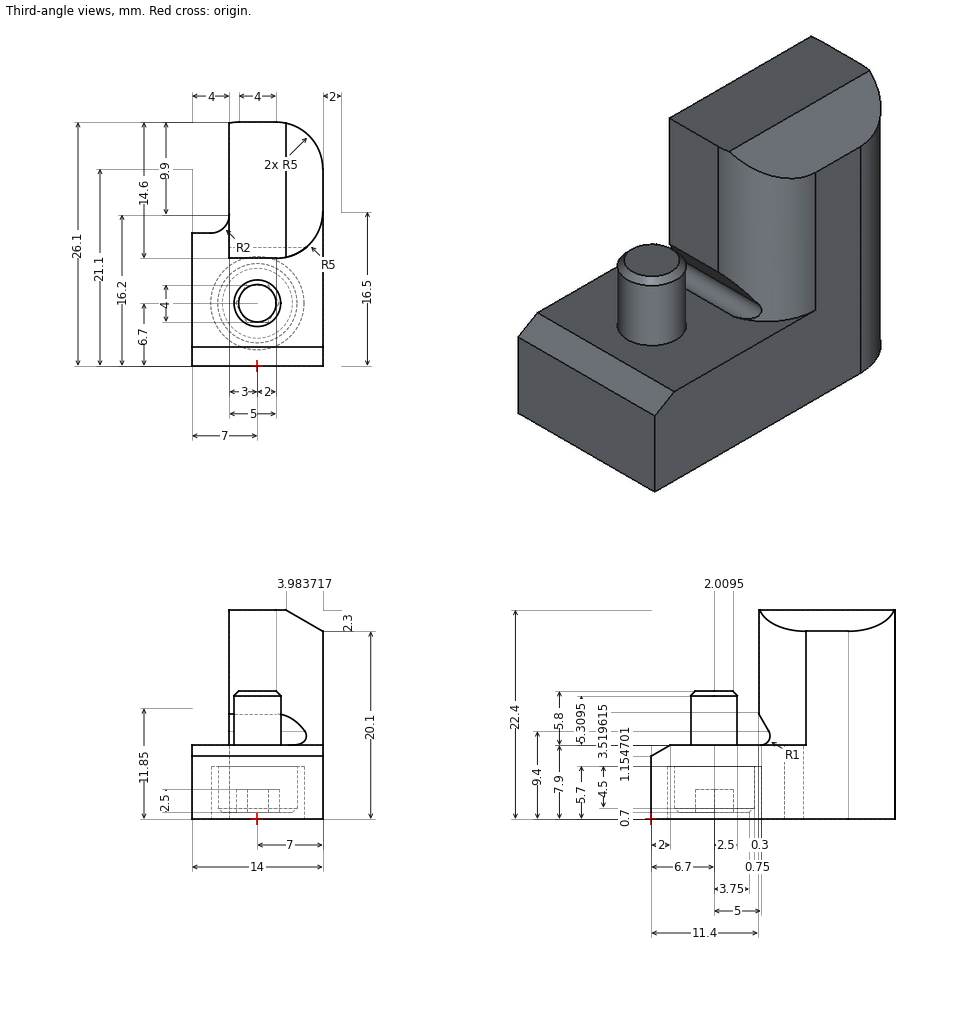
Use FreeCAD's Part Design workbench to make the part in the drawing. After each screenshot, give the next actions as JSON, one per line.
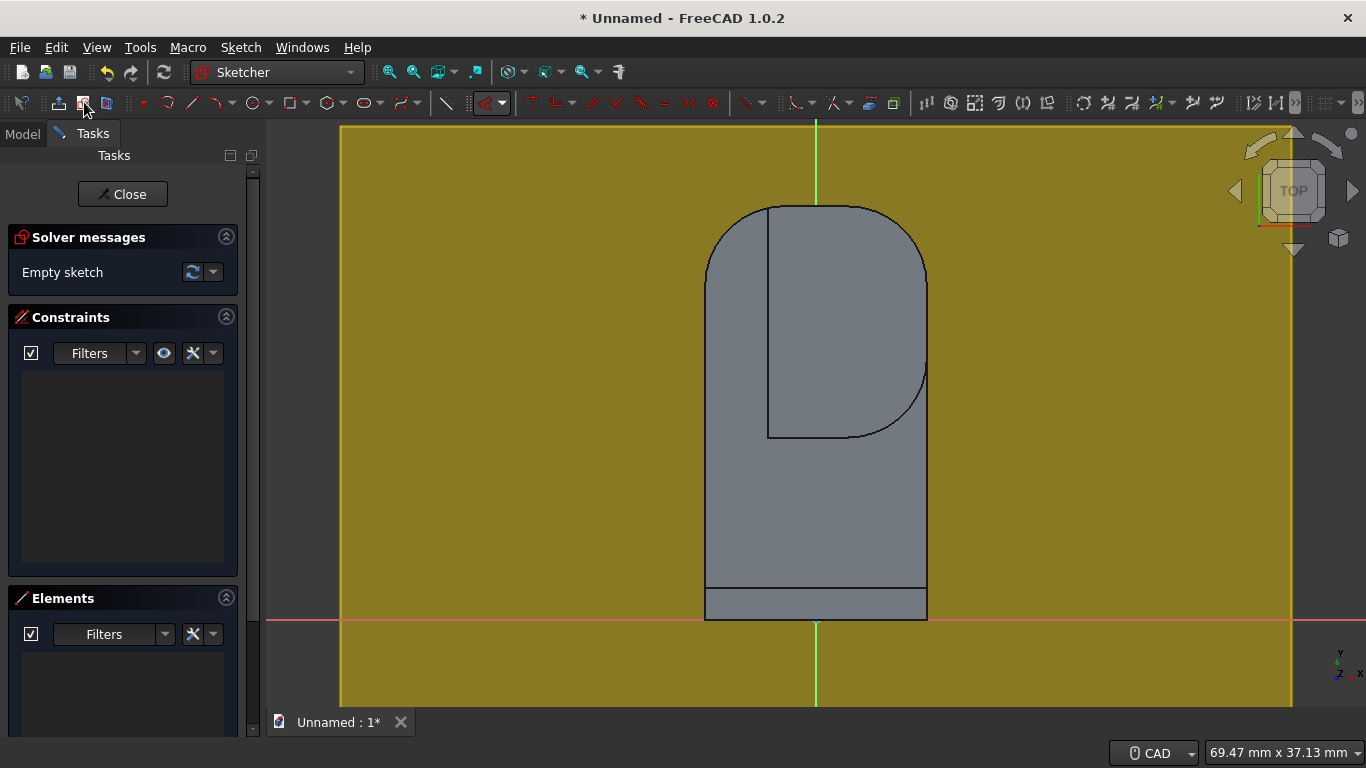
{"action": "left_click", "coordinate": [108, 104]}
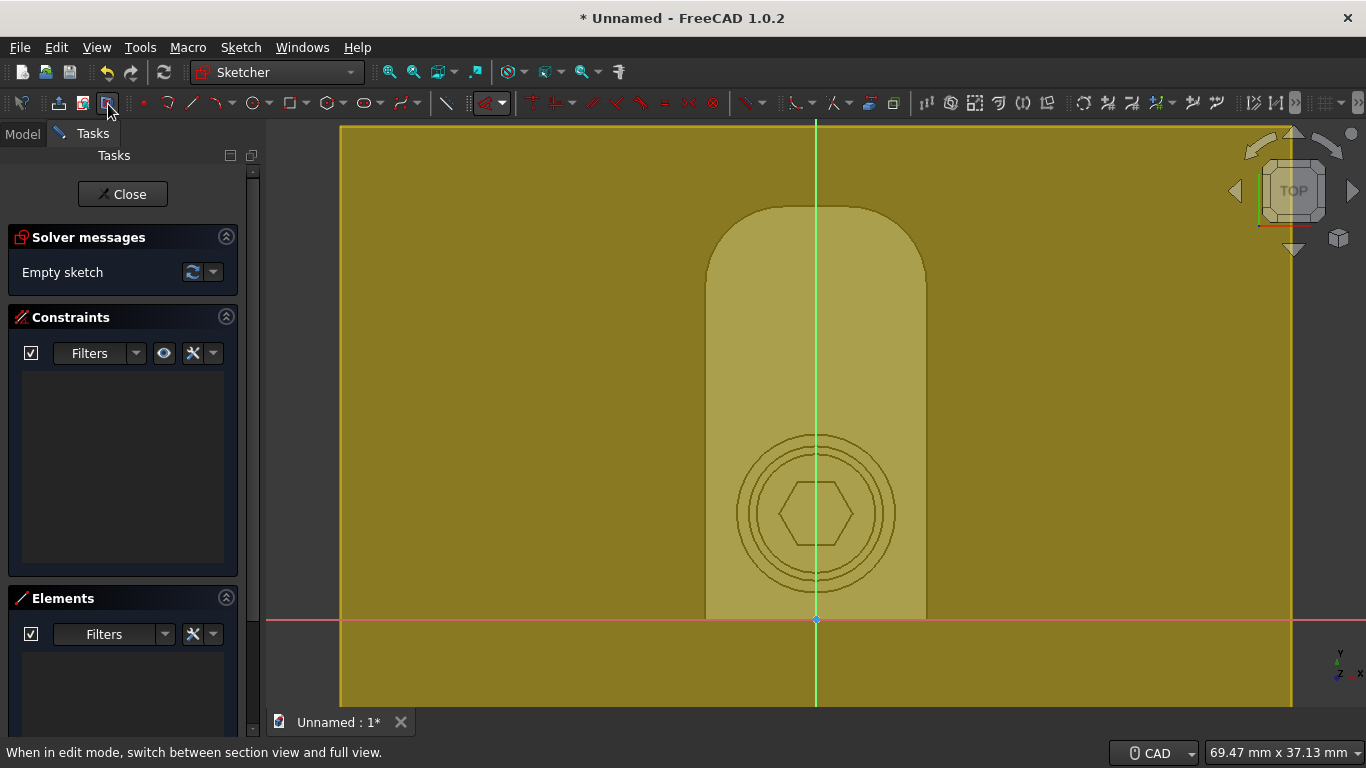
{"action": "left_click", "coordinate": [168, 104]}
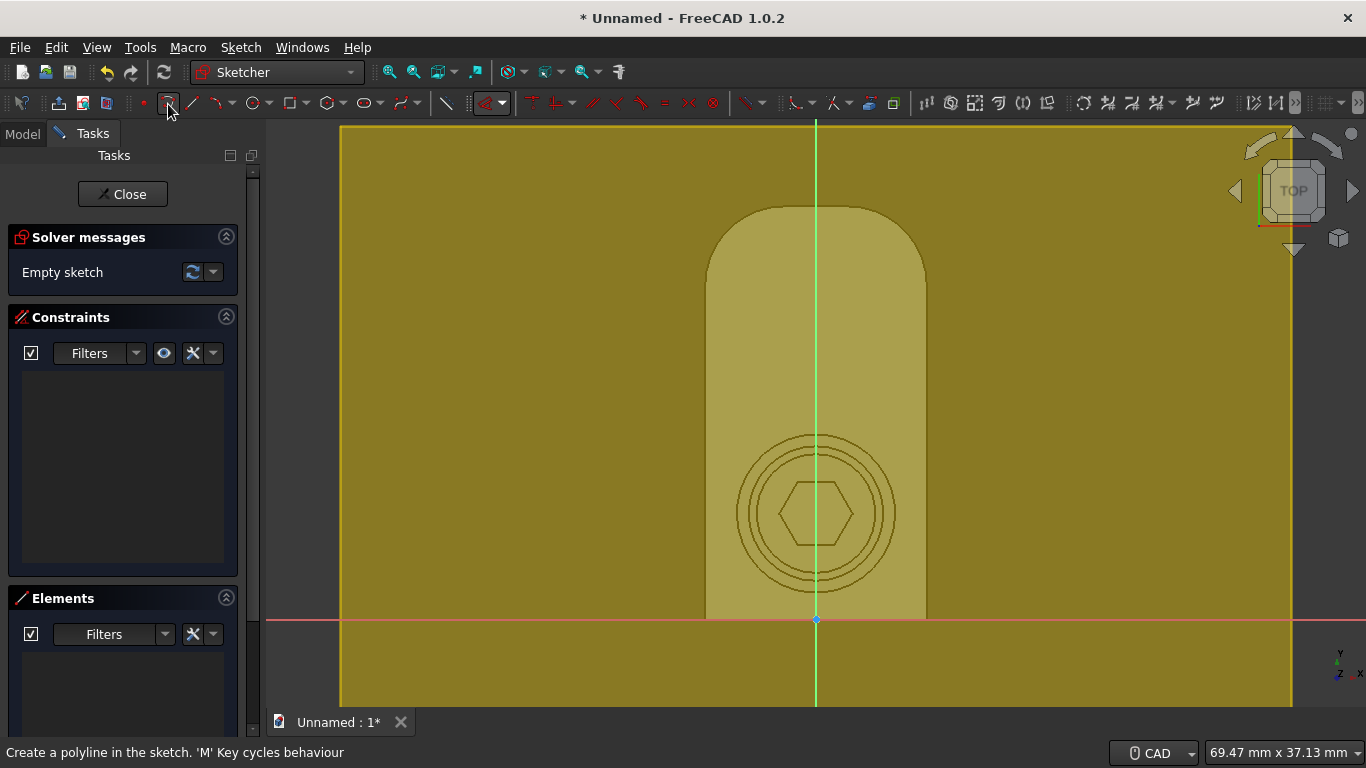
{"action": "left_click", "coordinate": [768, 363]}
{"action": "left_click", "coordinate": [768, 206]}
{"action": "left_click", "coordinate": [705, 206]}
{"action": "left_click", "coordinate": [705, 395]}
{"action": "left_click", "coordinate": [737, 395]}
{"action": "right_click", "coordinate": [737, 395]}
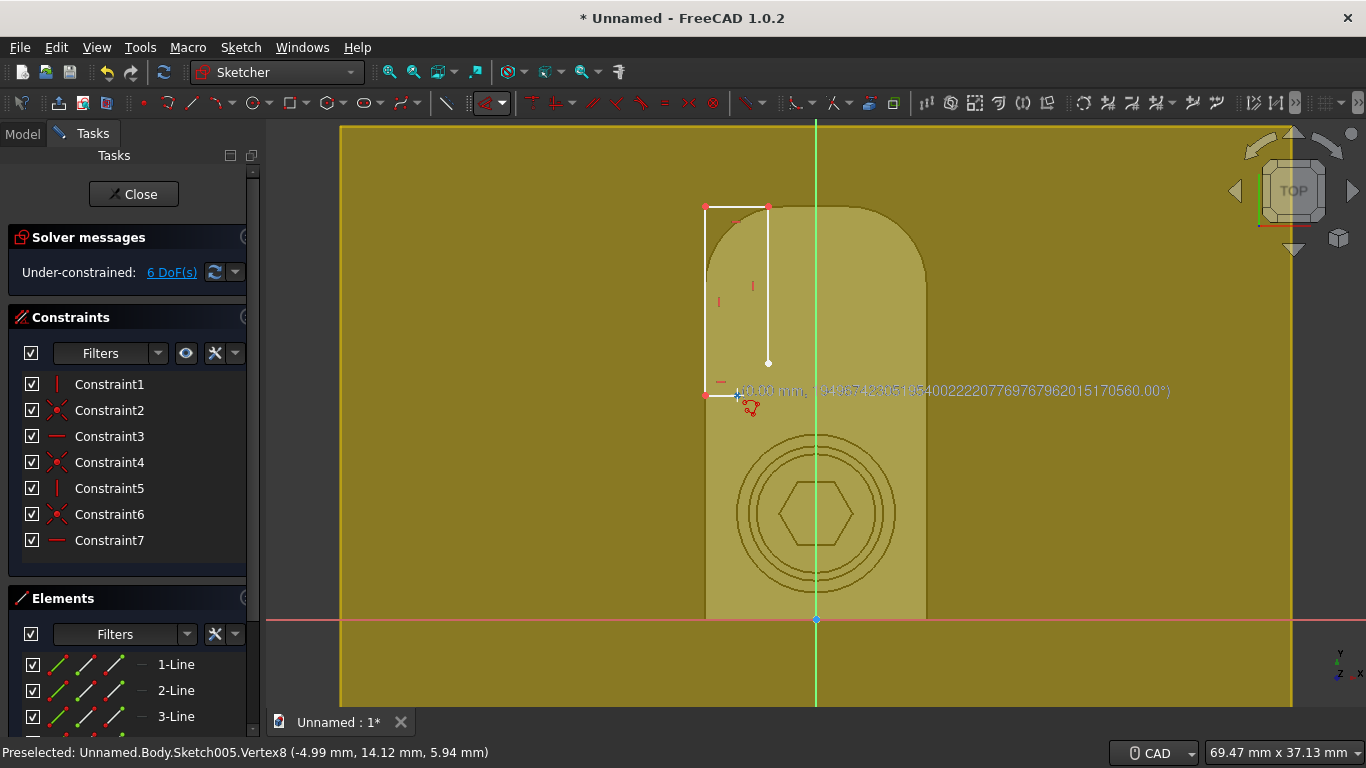
{"action": "left_click", "coordinate": [216, 104]}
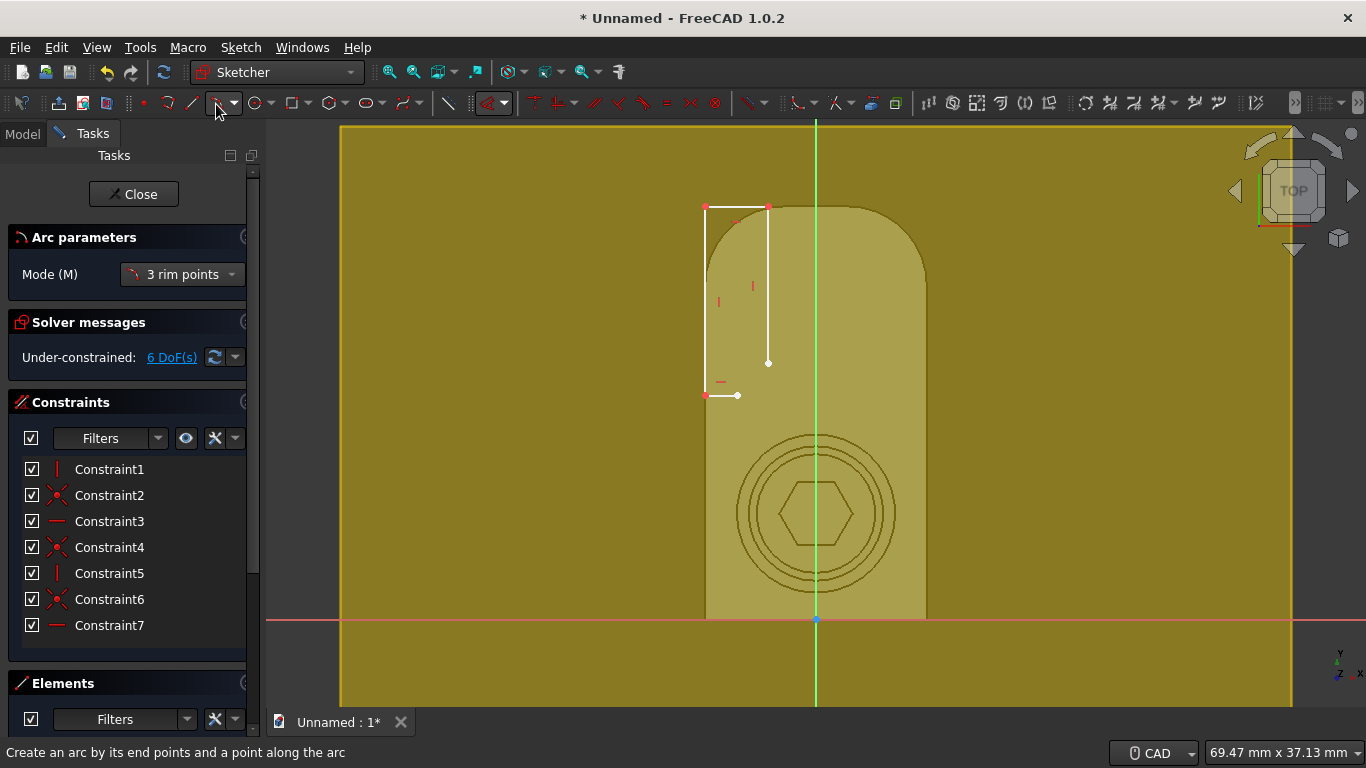
{"action": "left_click", "coordinate": [737, 396]}
{"action": "left_click", "coordinate": [768, 364]}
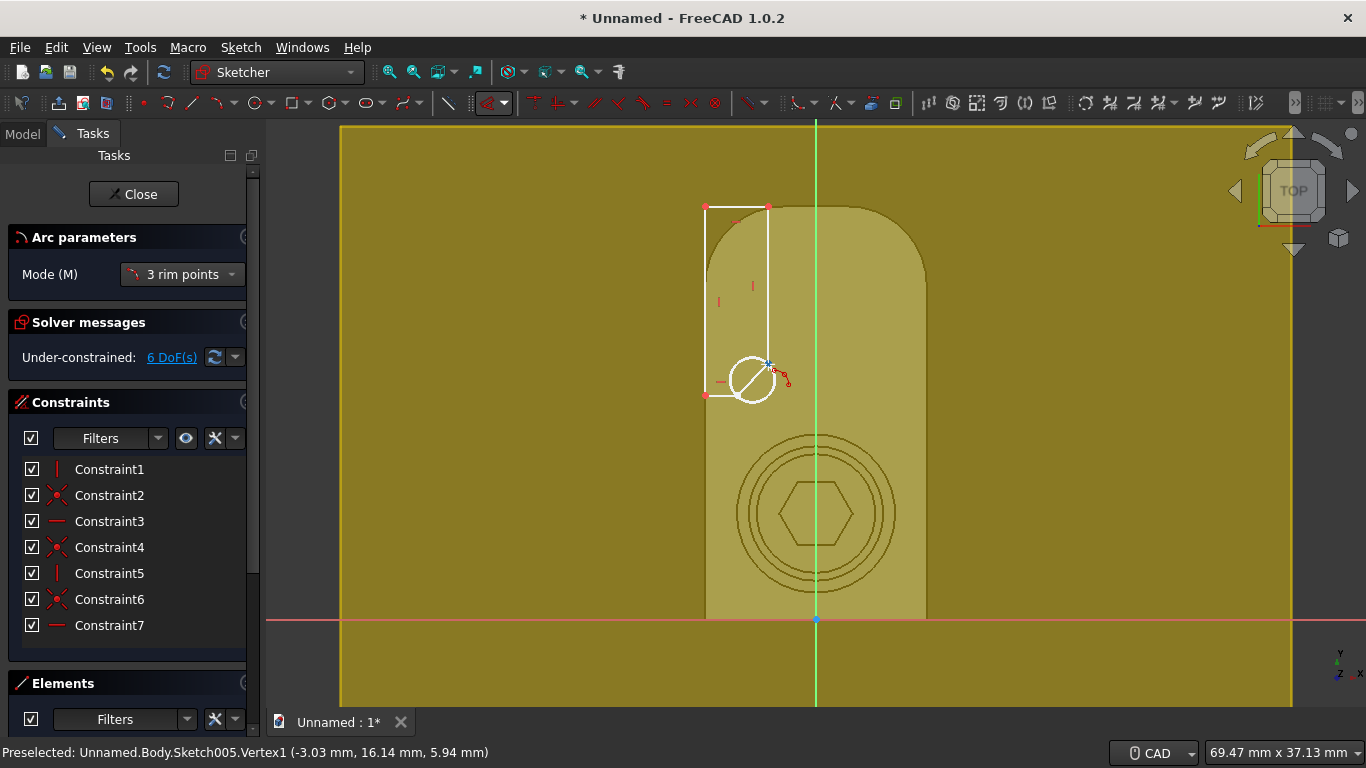
{"action": "scroll", "coordinate": [759, 386], "scroll_direction": "up", "scroll_amount": 3}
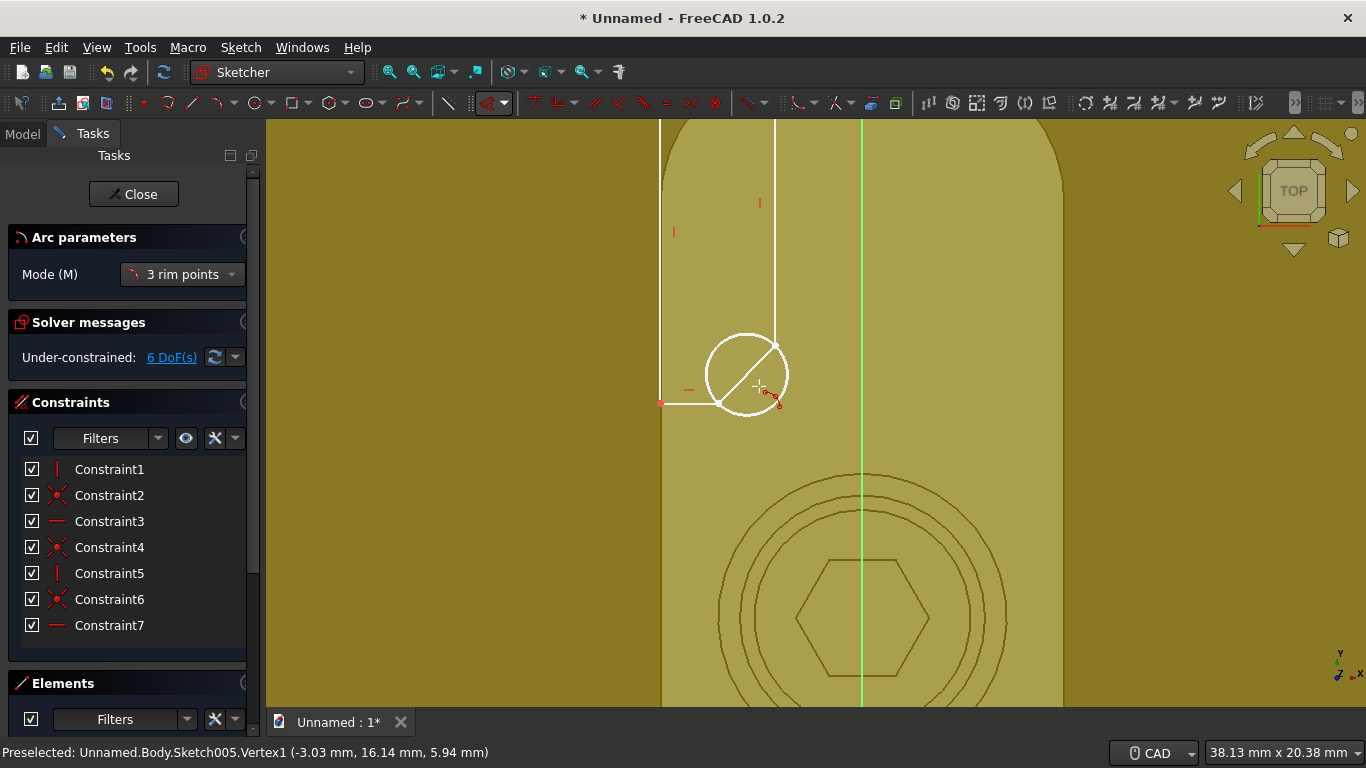
{"action": "left_click", "coordinate": [759, 385]}
{"action": "key", "text": "Escape"}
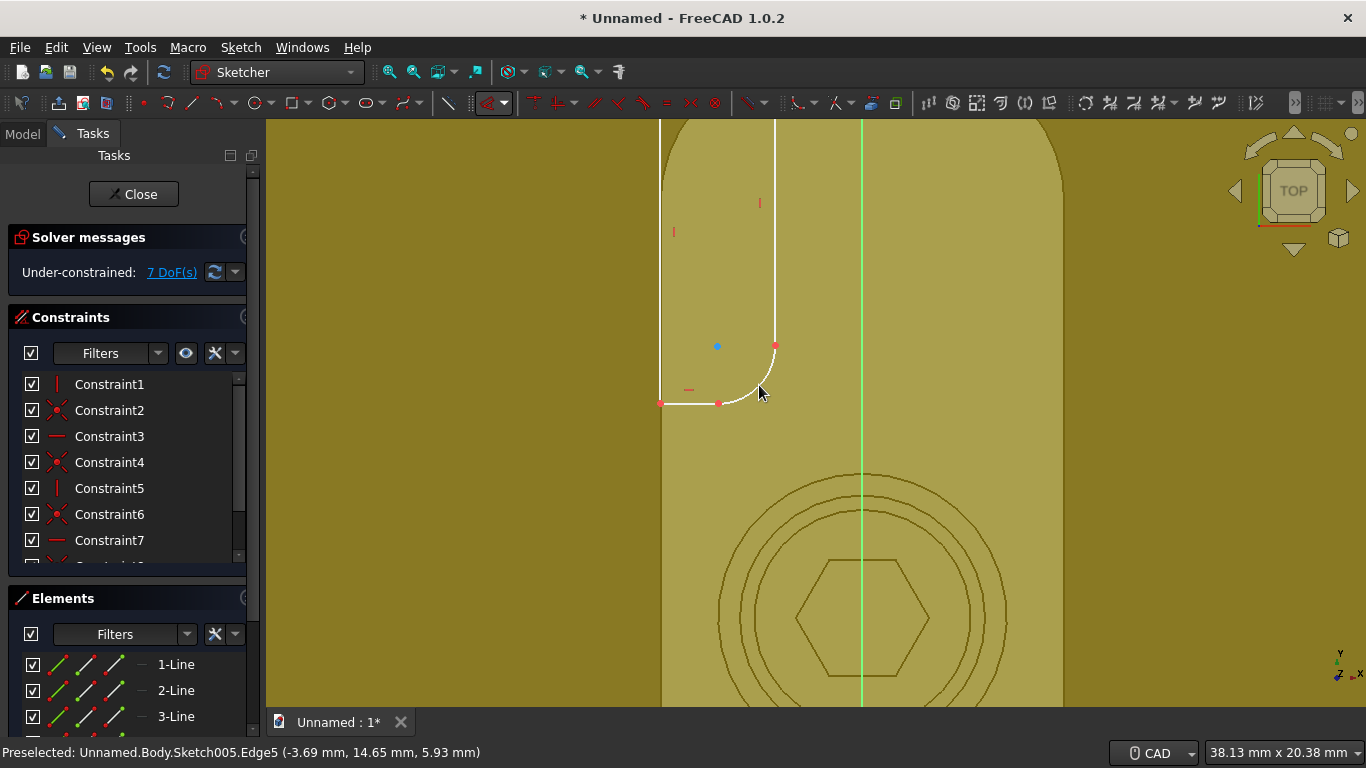
{"action": "left_click", "coordinate": [775, 260]}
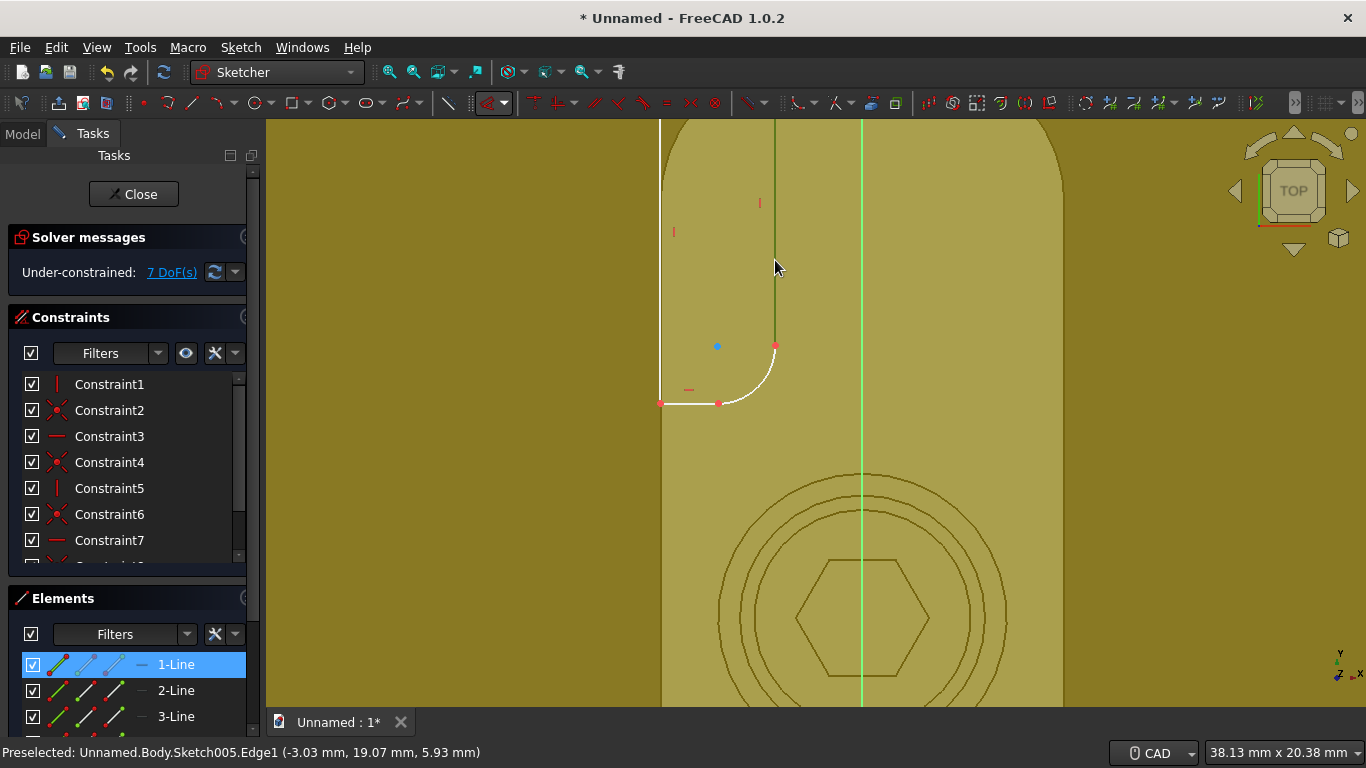
{"action": "left_click", "coordinate": [744, 397]}